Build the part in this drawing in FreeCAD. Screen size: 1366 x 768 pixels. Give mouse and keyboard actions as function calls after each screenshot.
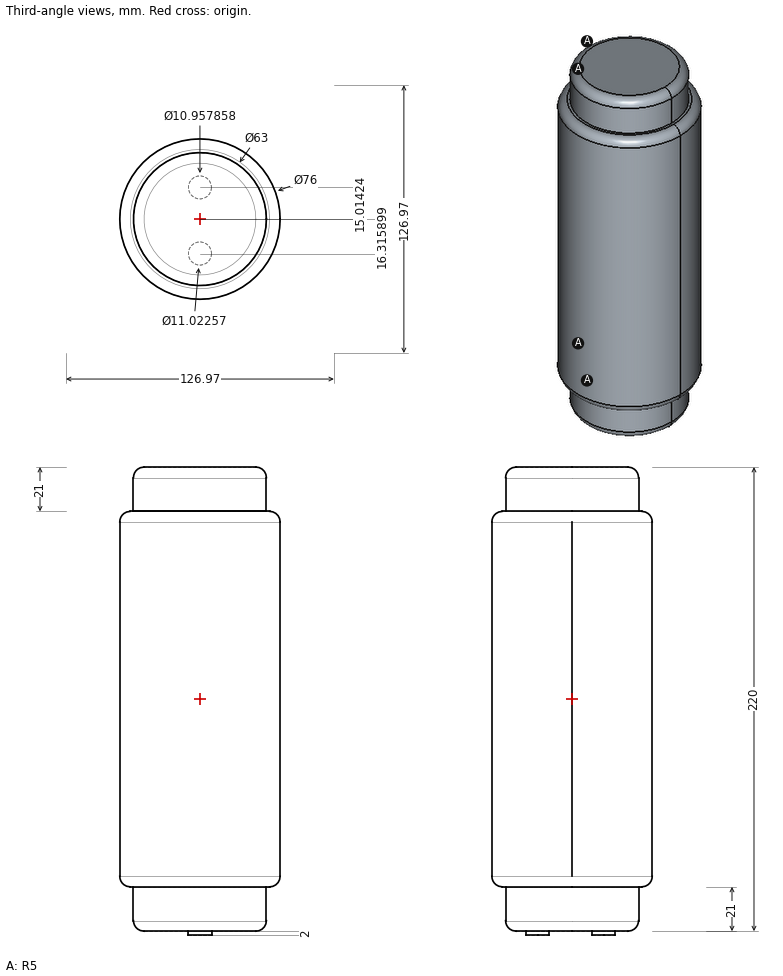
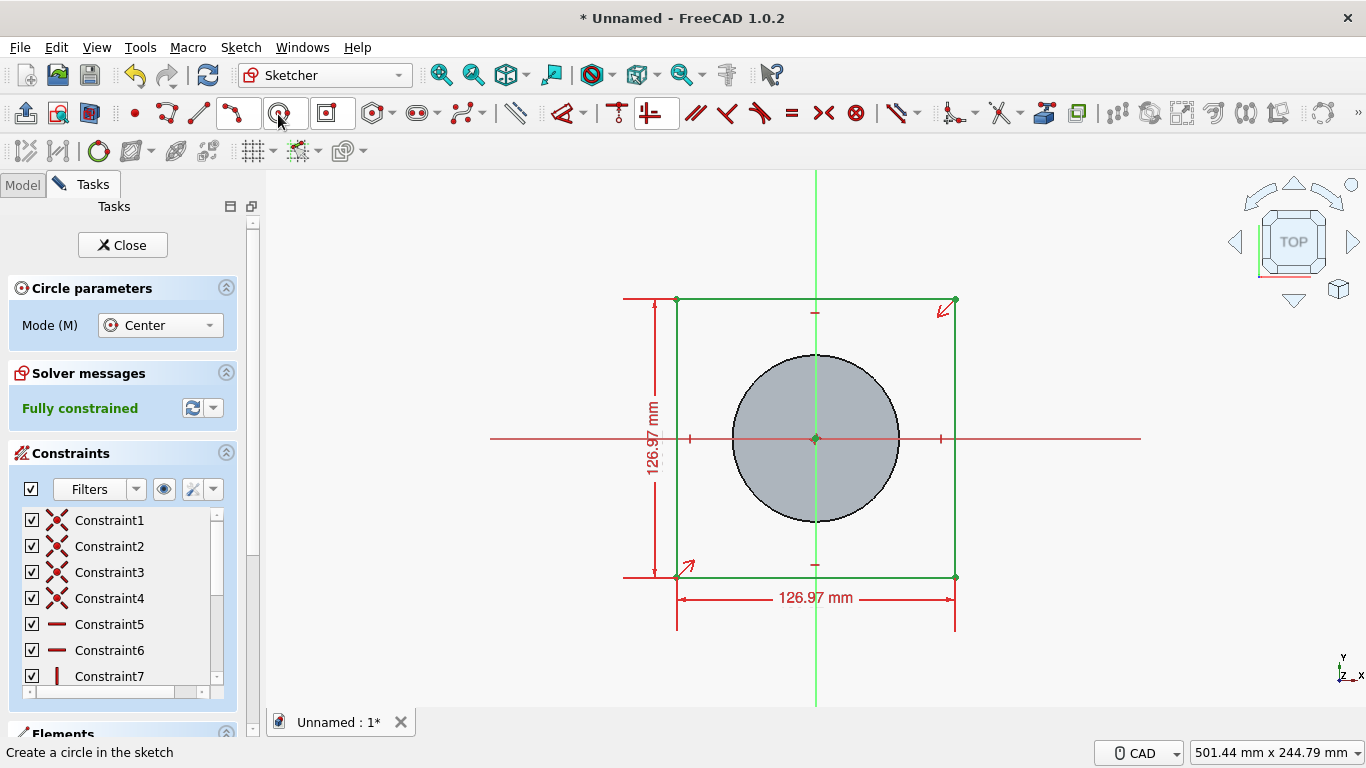
click(816, 438)
move(865, 390)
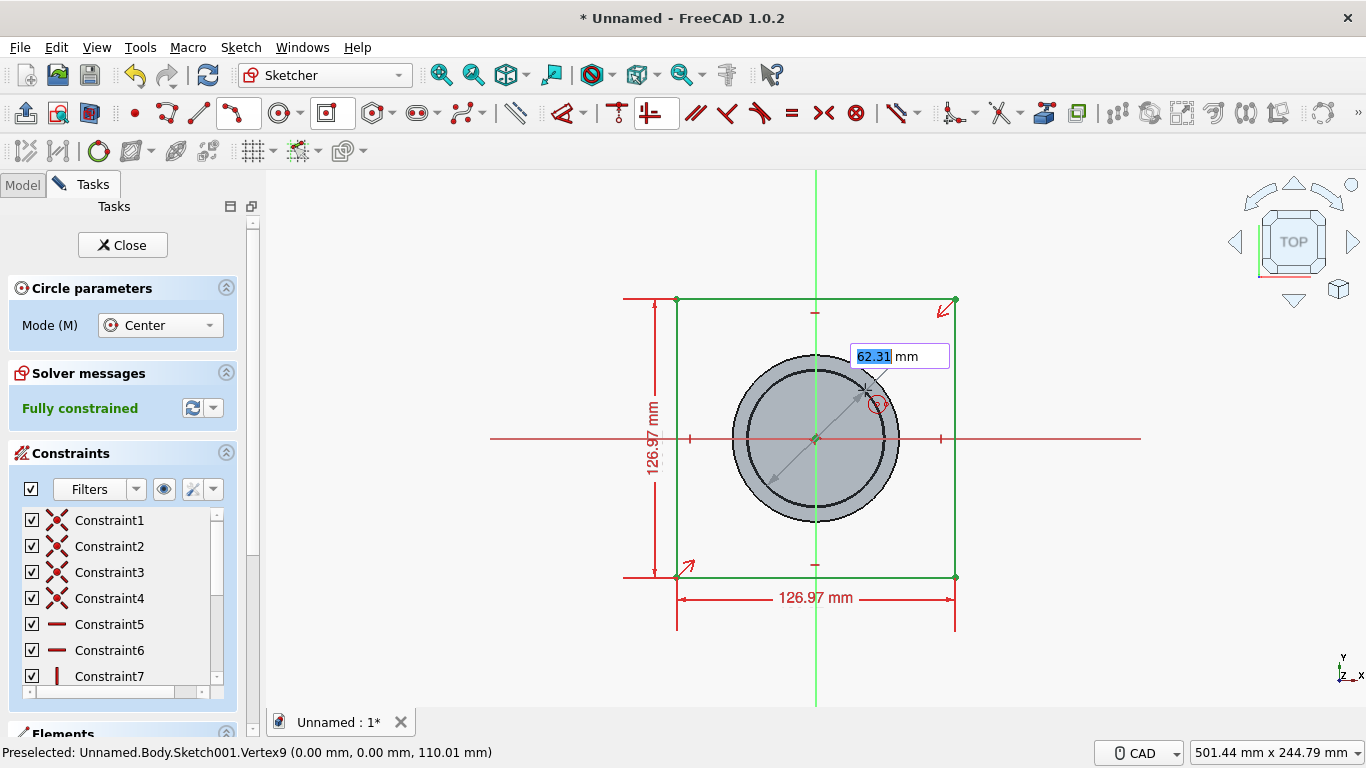
text(63)
key(Return)
key(Escape)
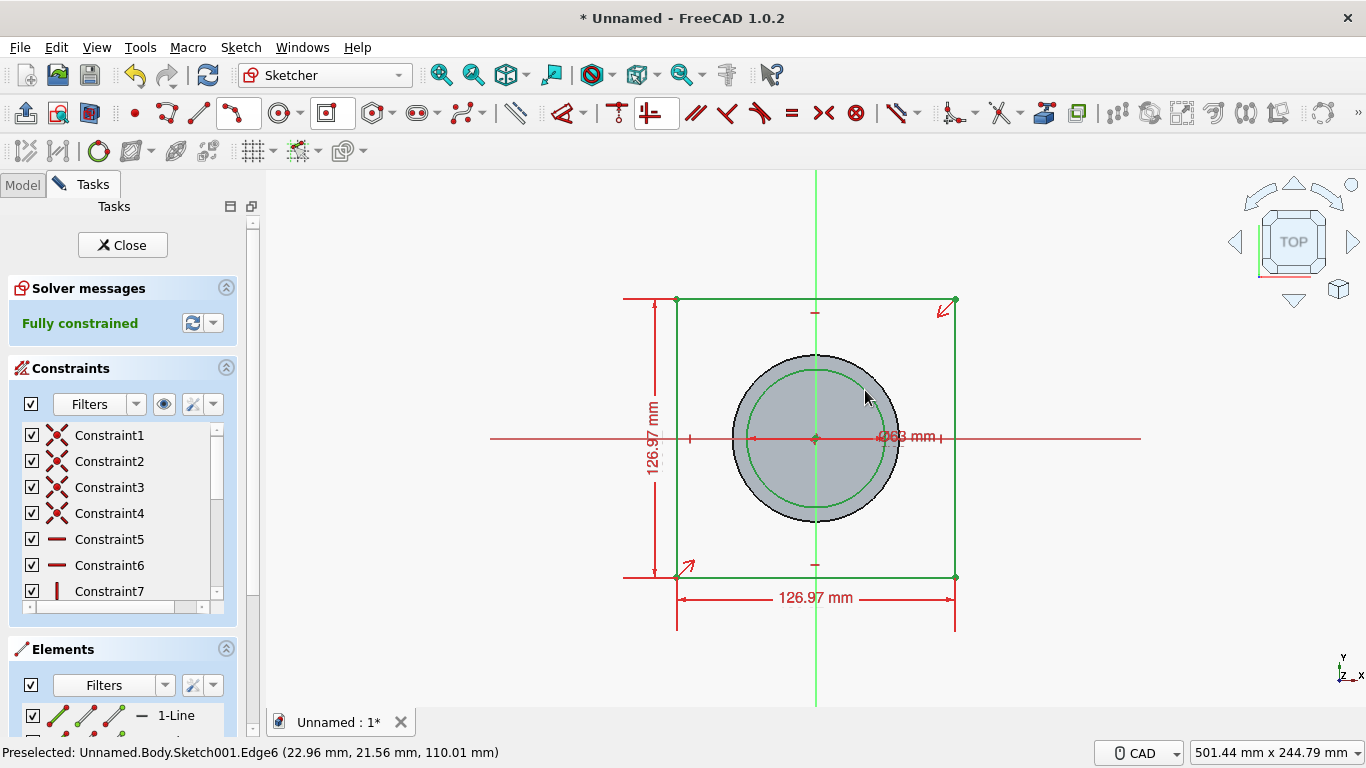
click(123, 245)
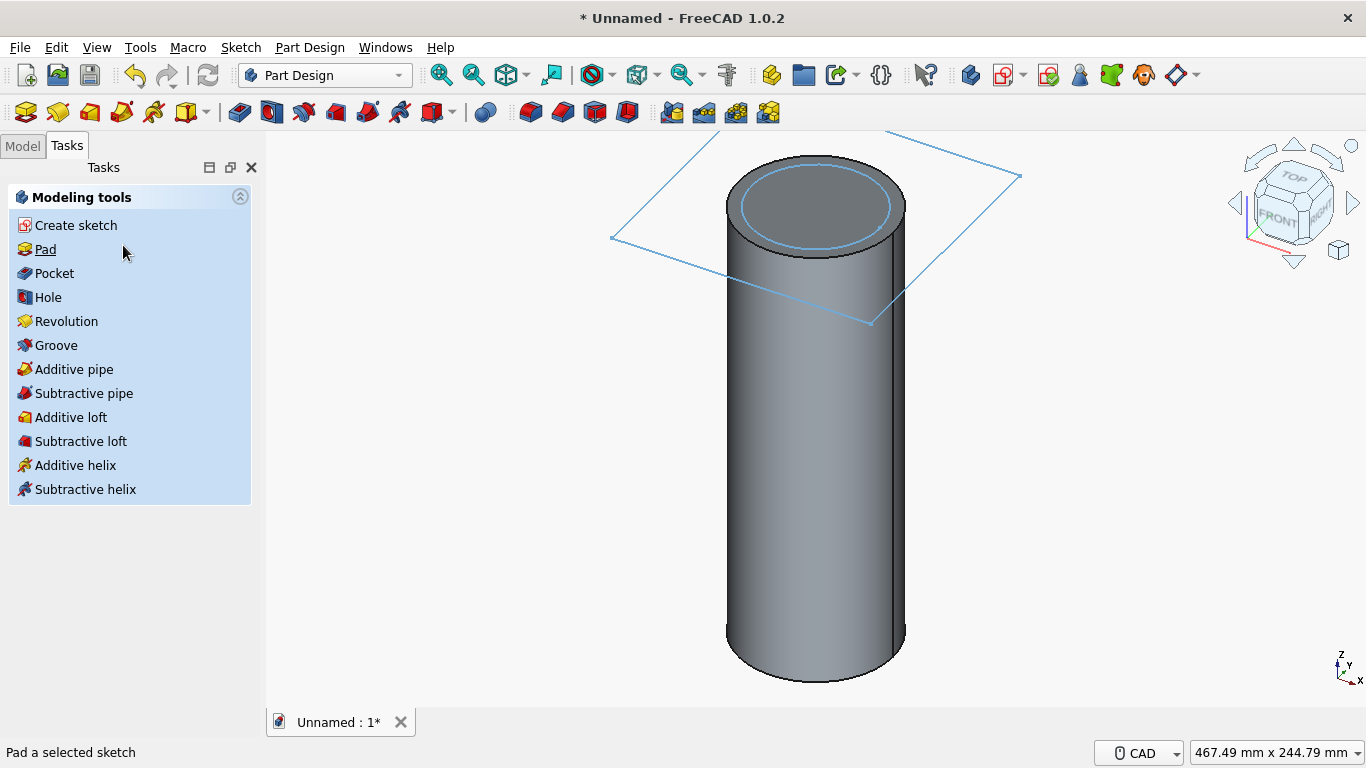
click(240, 112)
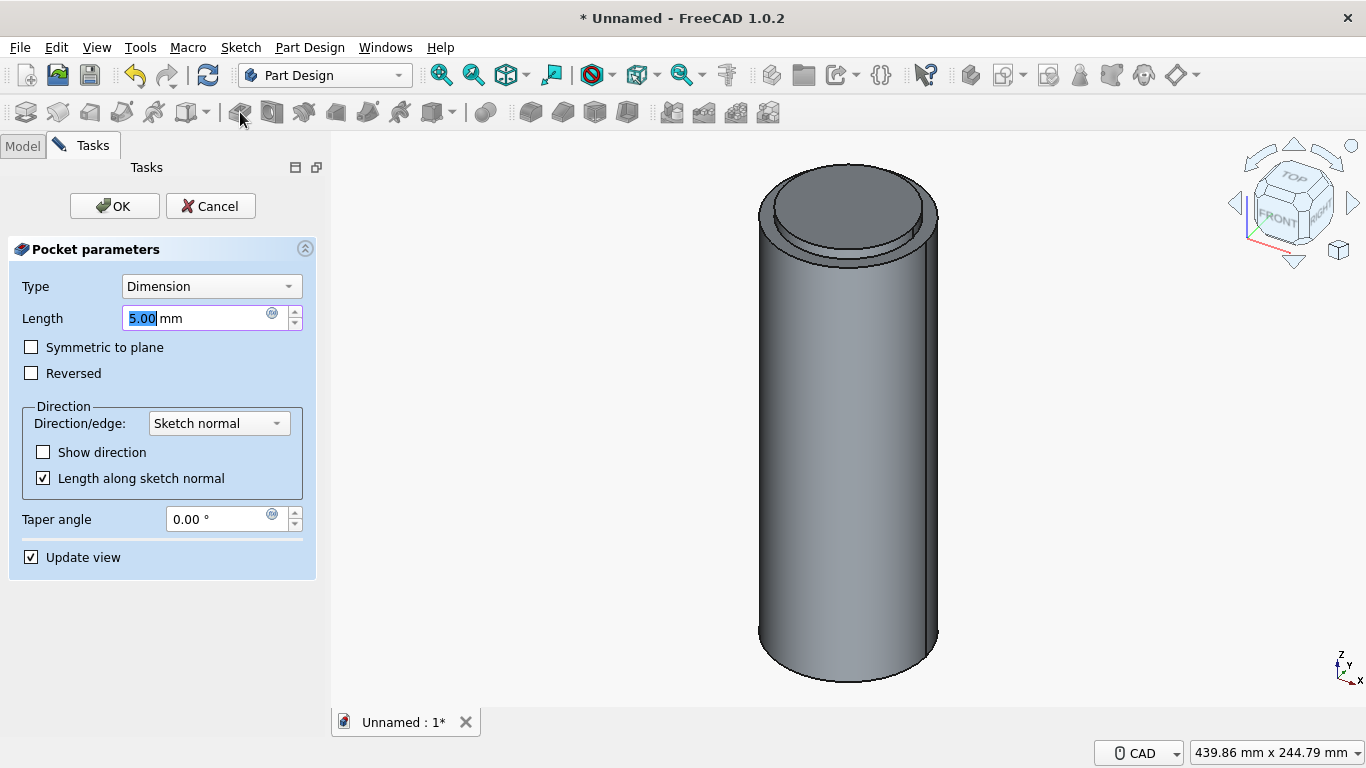
text(21)
key(Tab)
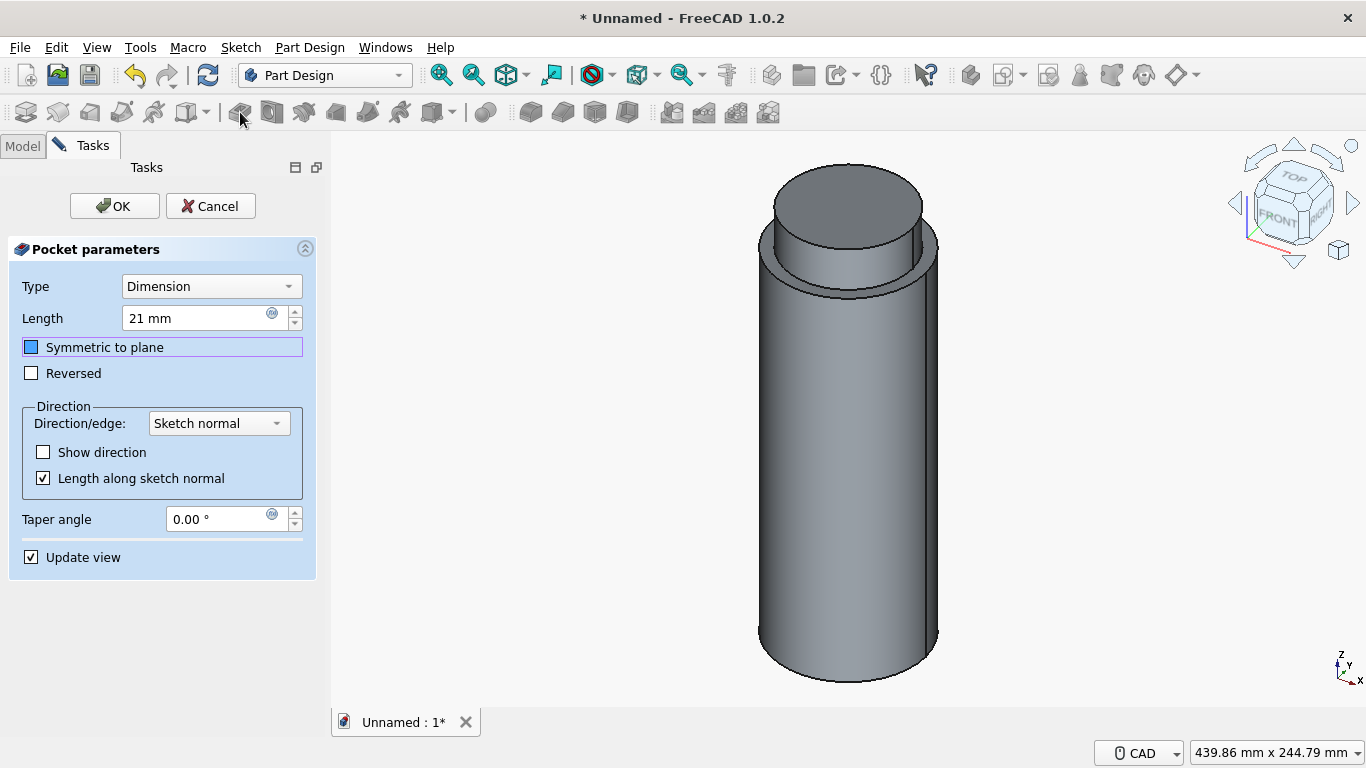
click(115, 206)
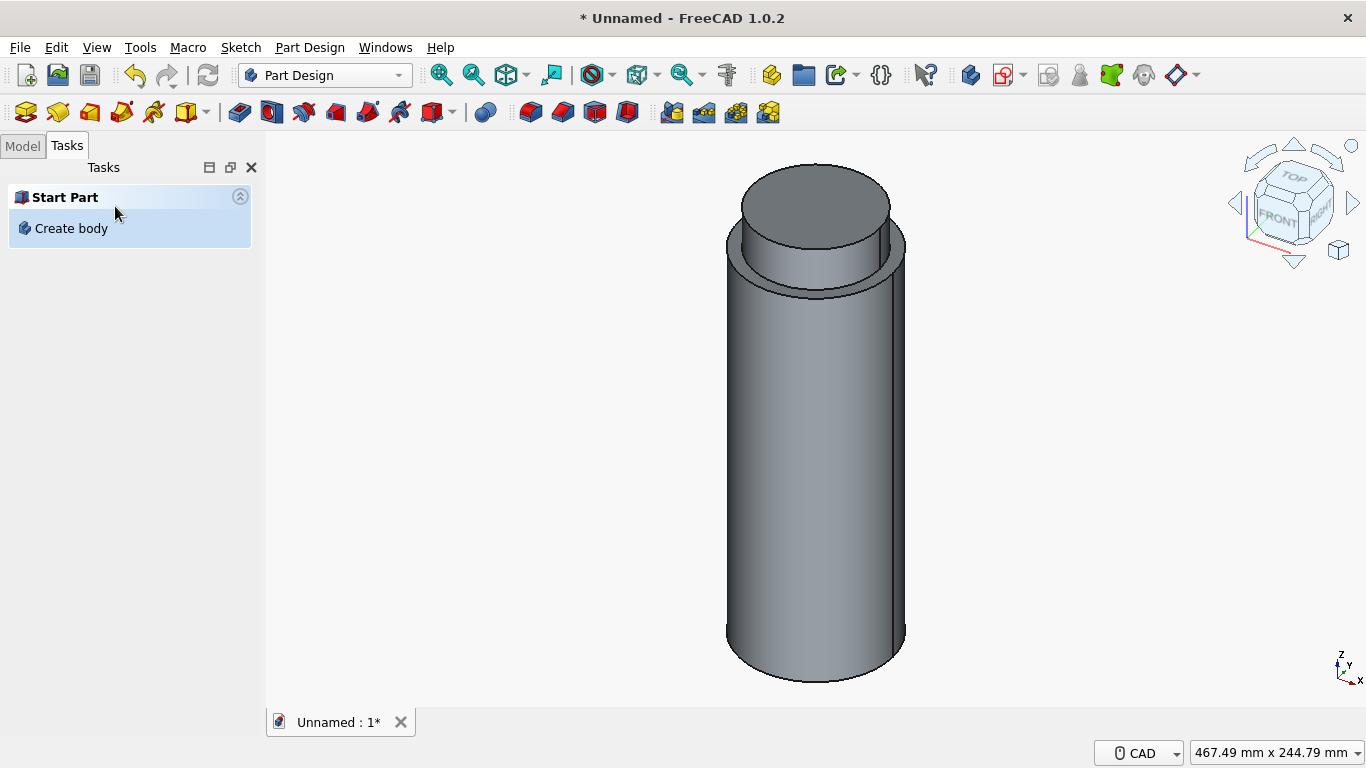
key(5)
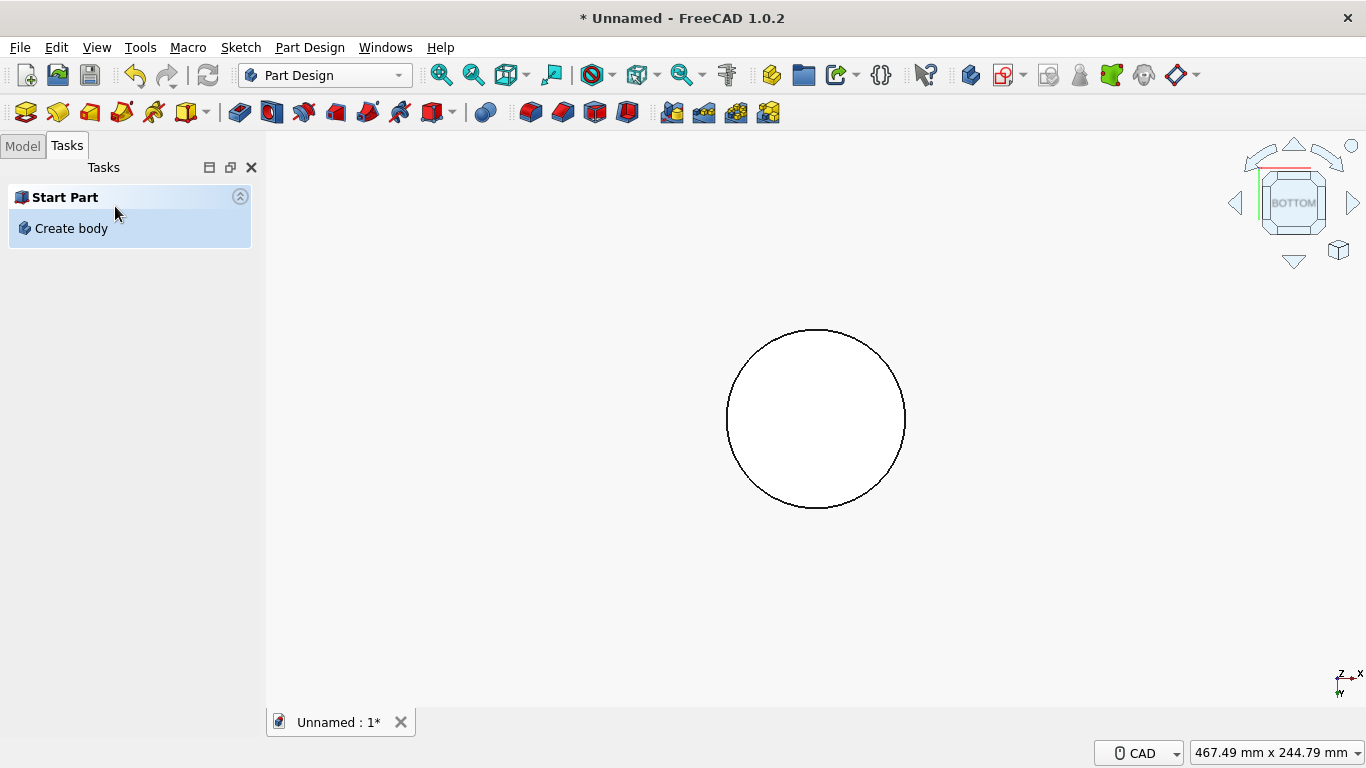
click(442, 76)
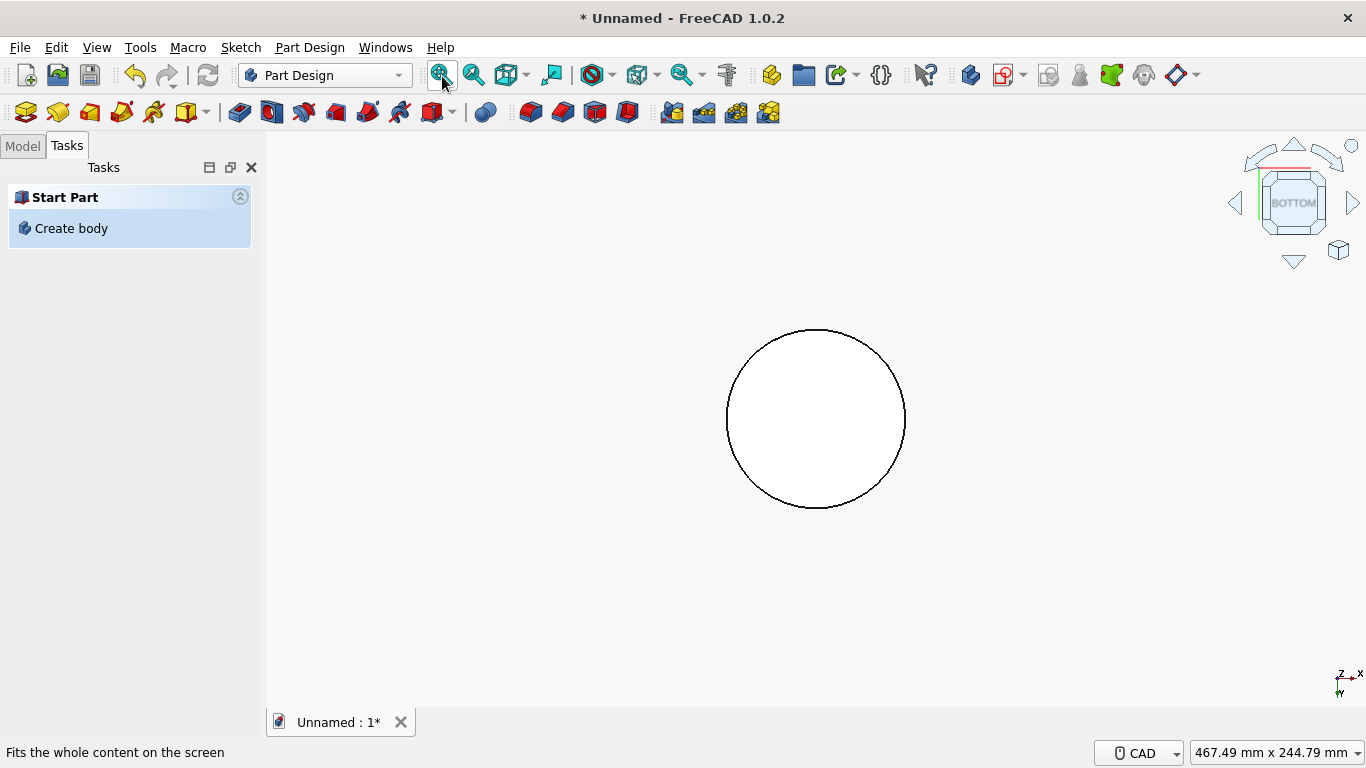
click(816, 418)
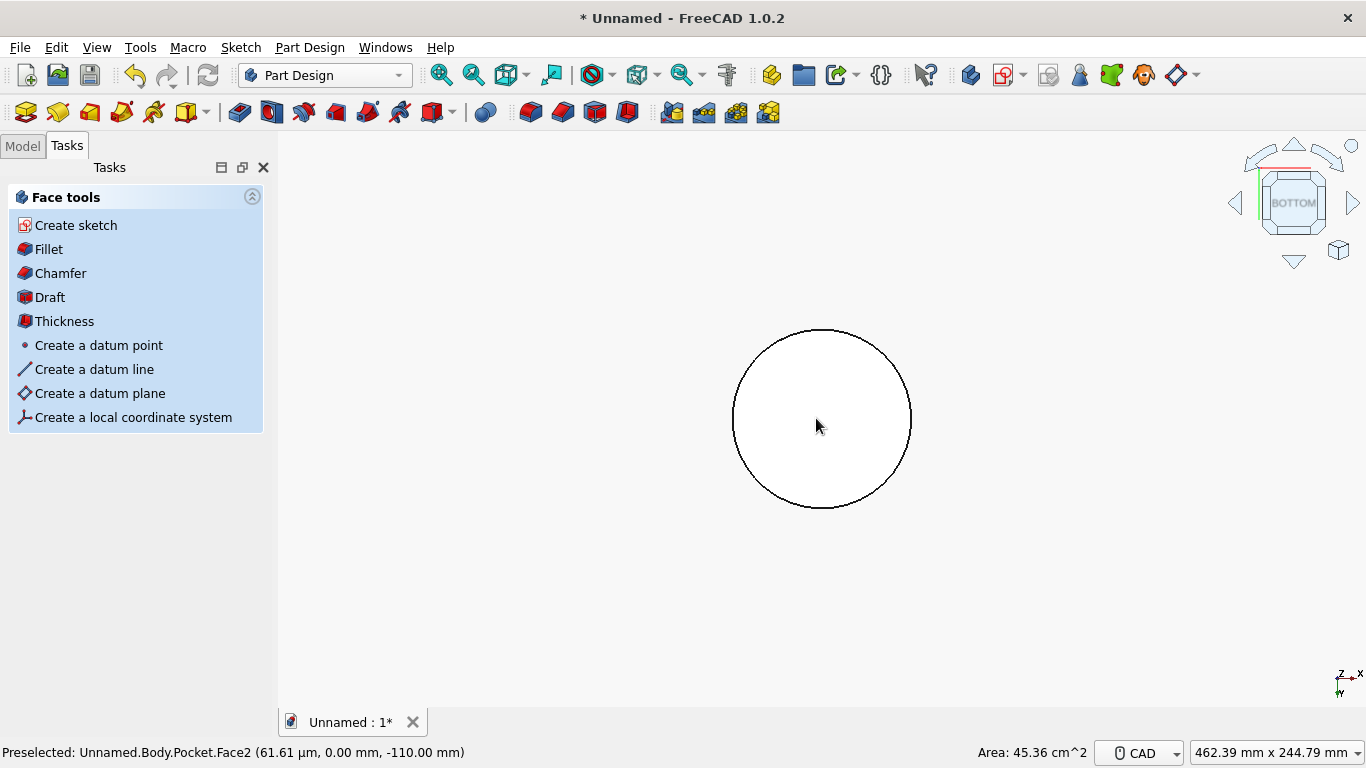
click(1004, 76)